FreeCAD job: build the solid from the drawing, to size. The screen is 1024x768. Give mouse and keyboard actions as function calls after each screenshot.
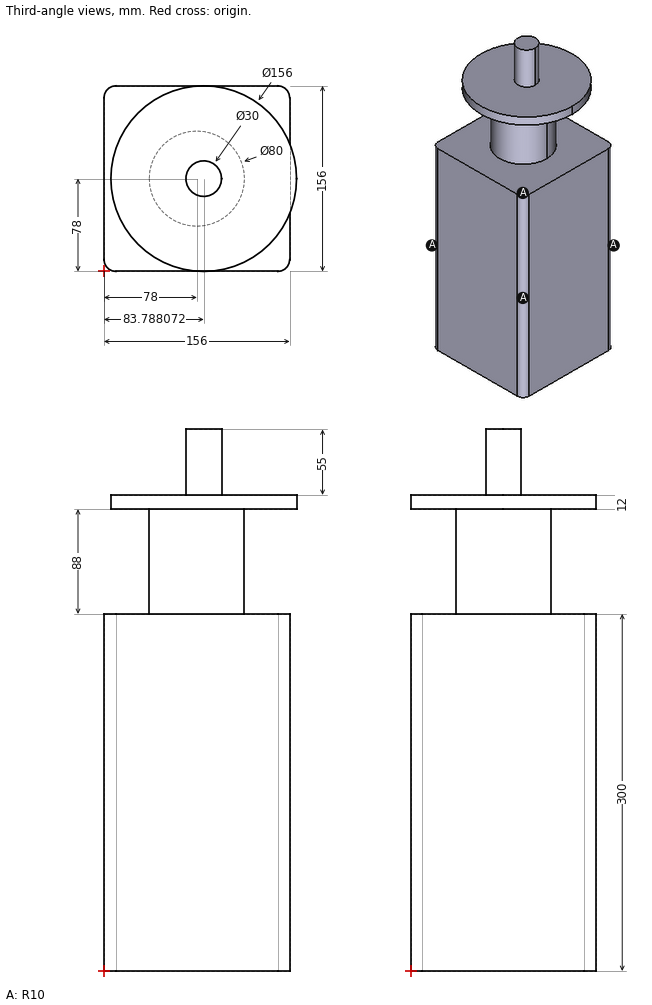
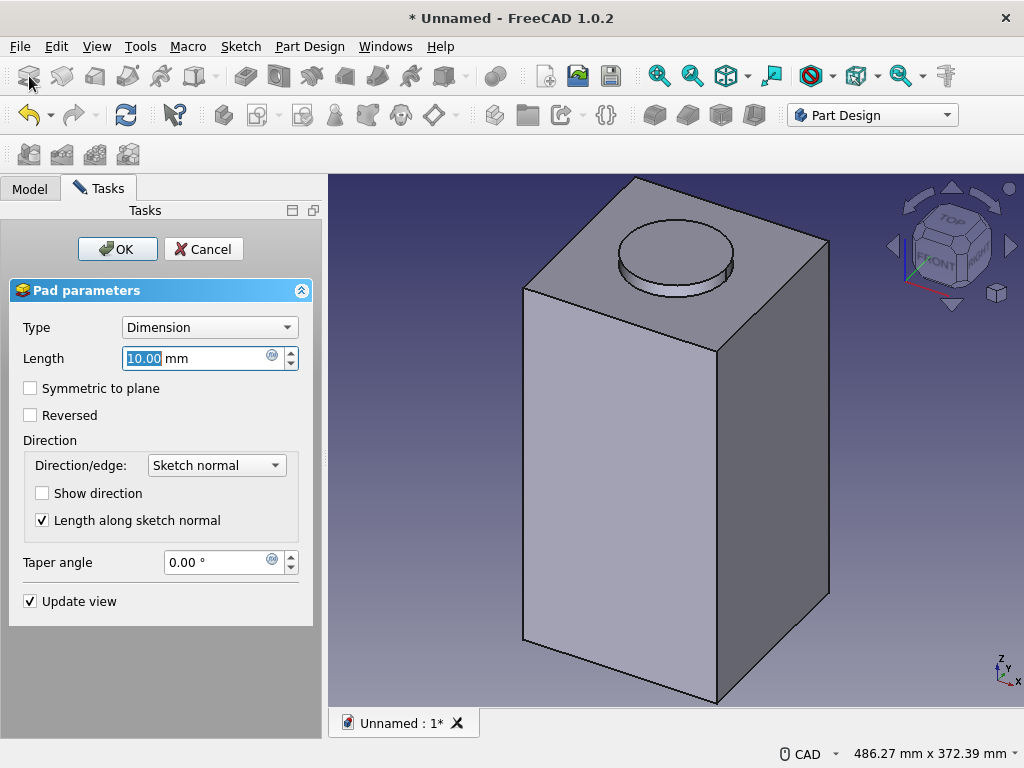
text(88)
key(Tab)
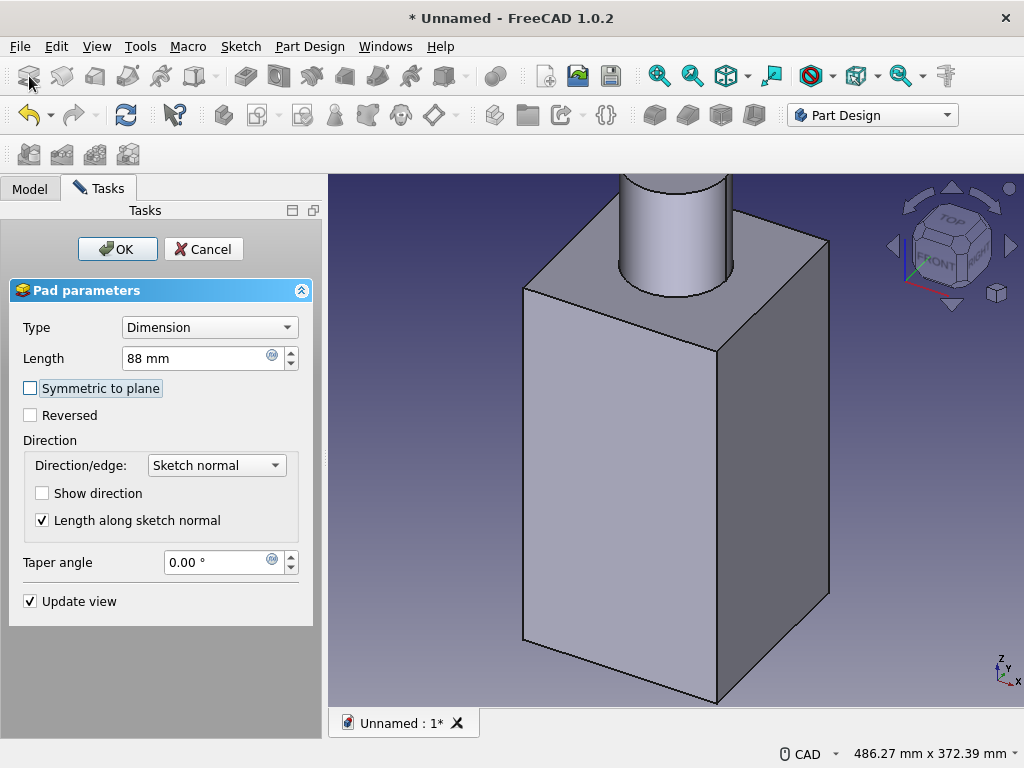
click(118, 249)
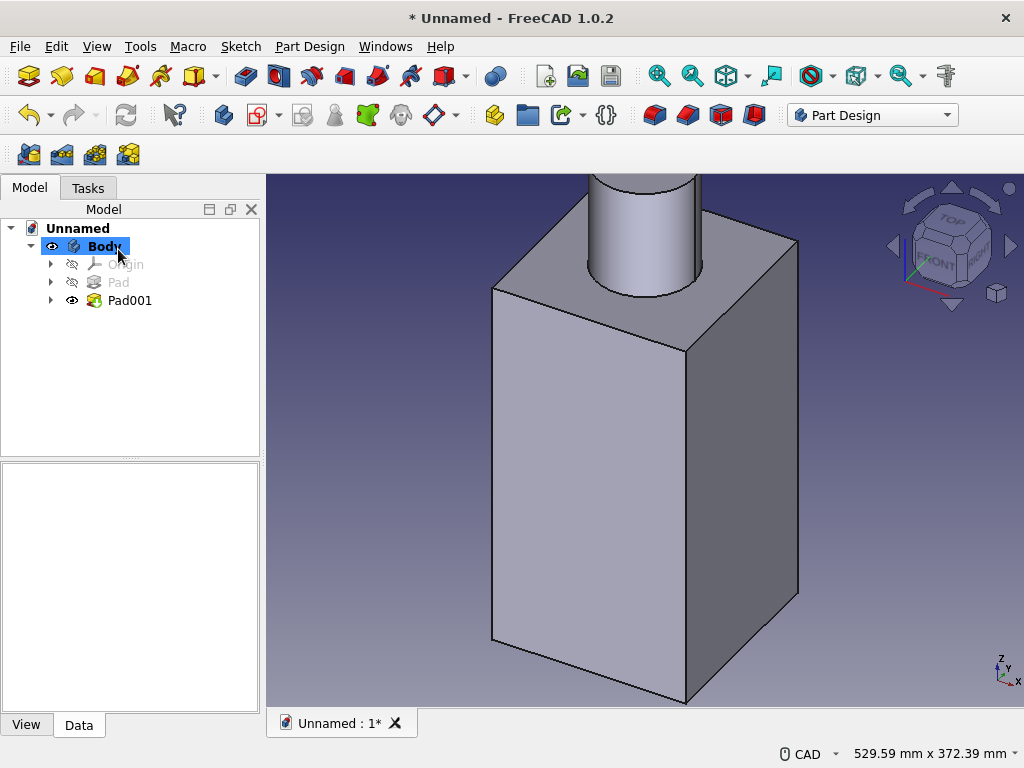
click(660, 76)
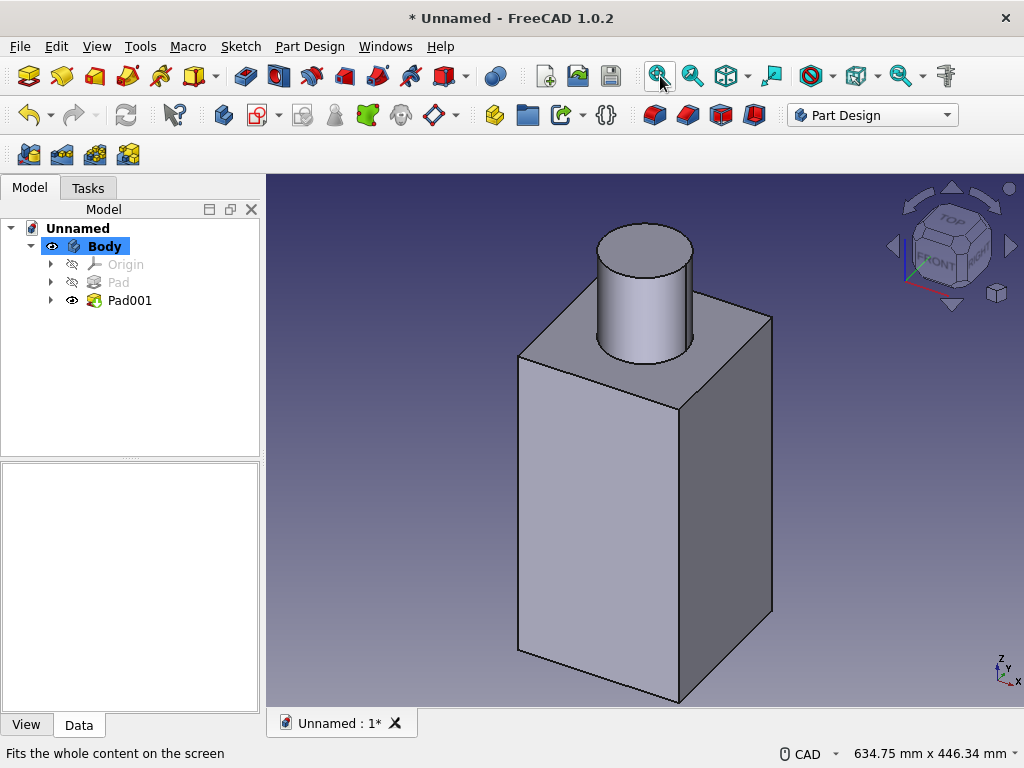
click(645, 250)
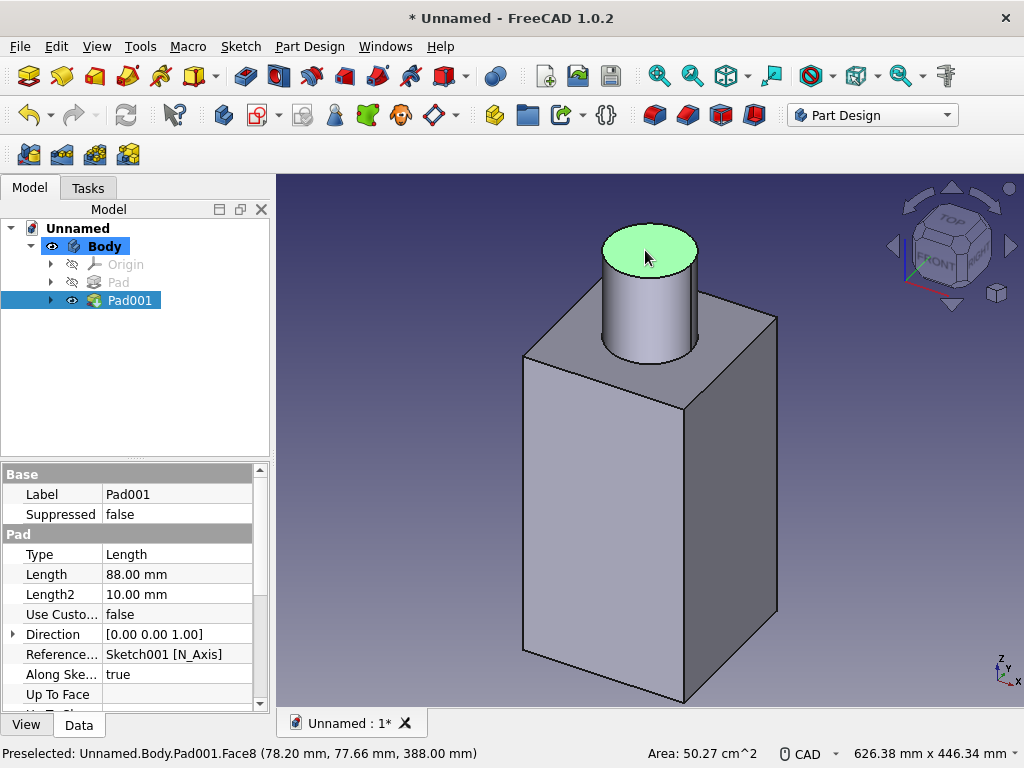
click(256, 116)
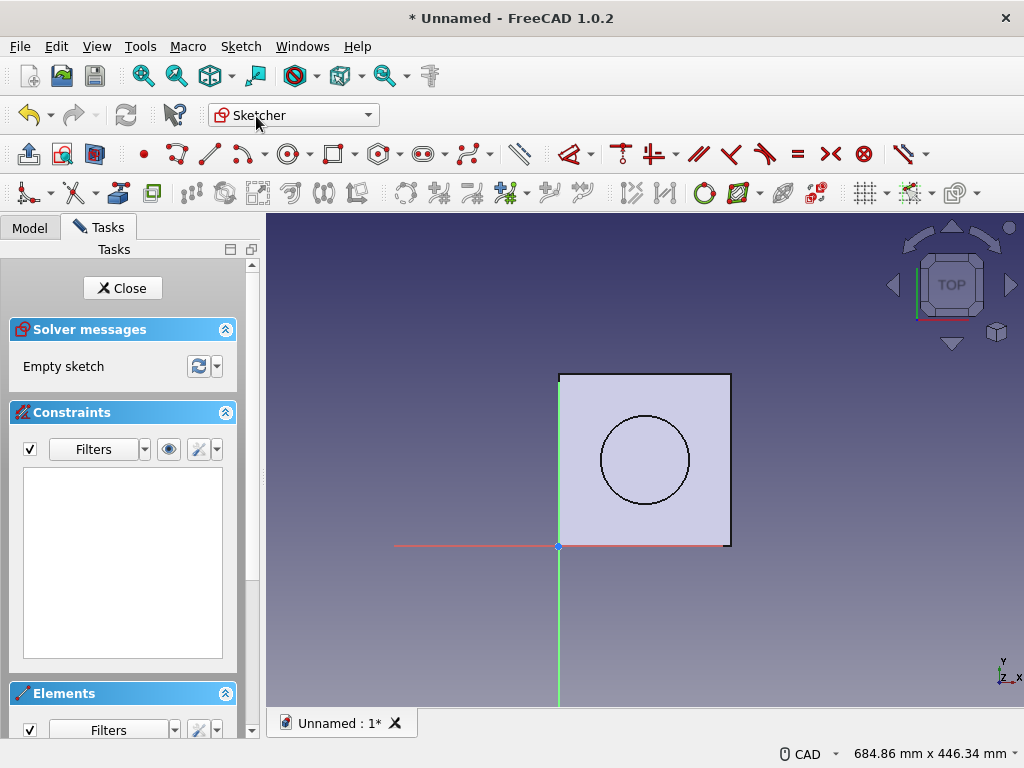
scroll(735, 460, up, 3)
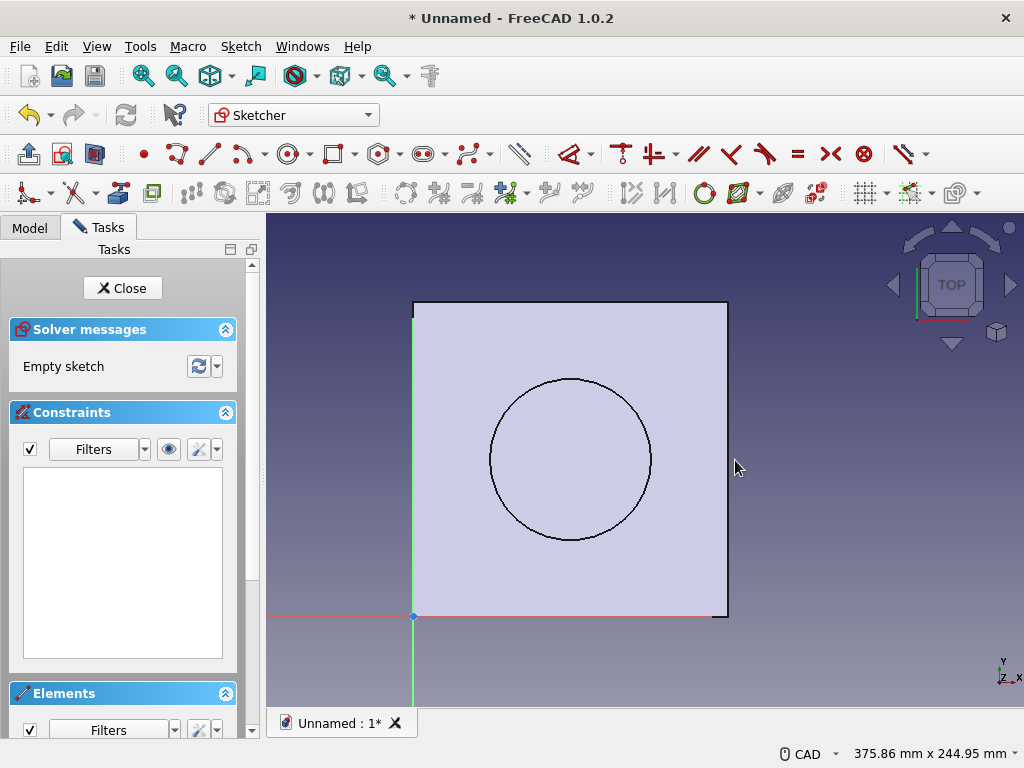
click(288, 154)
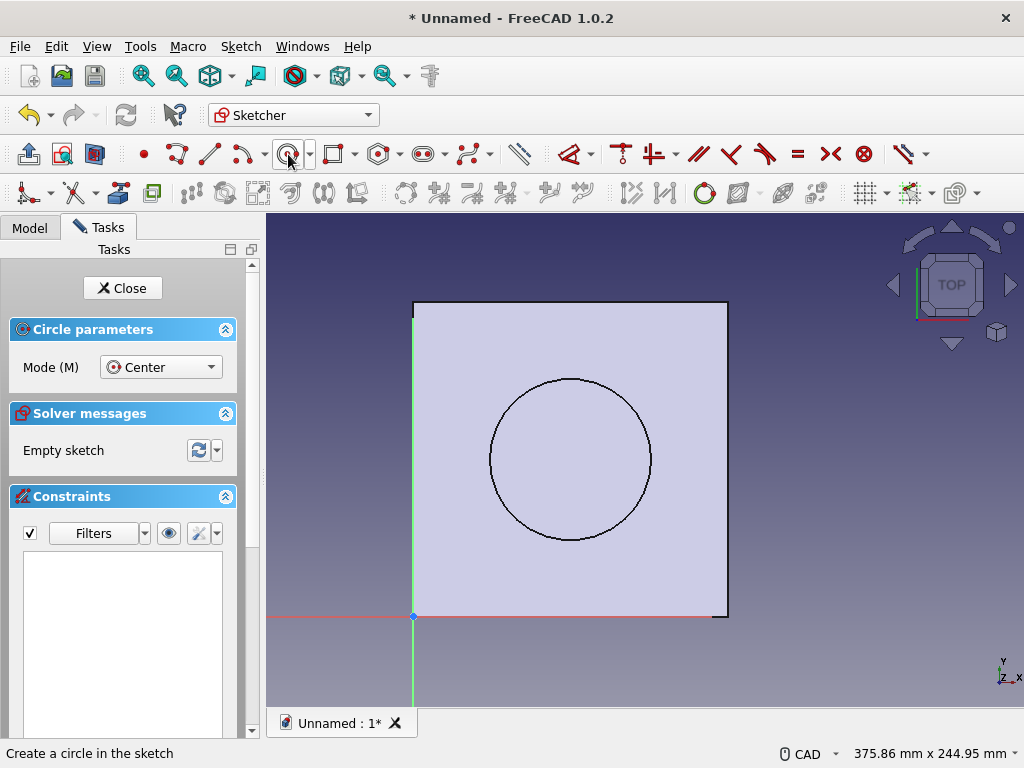
click(582, 460)
move(693, 348)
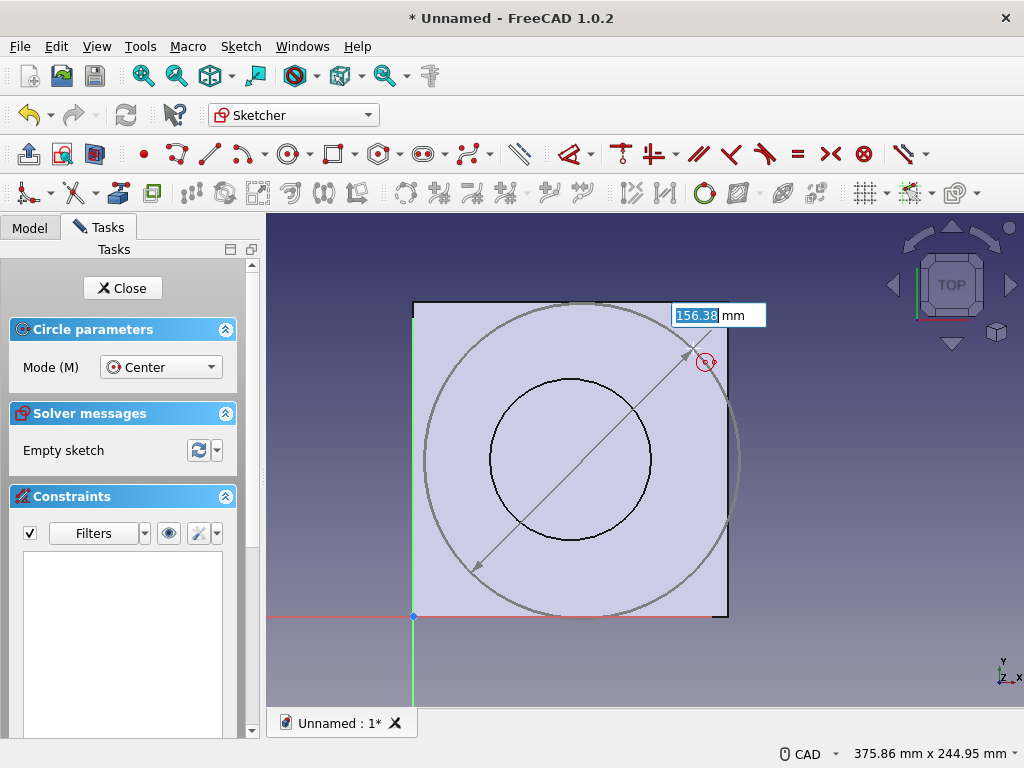
text(156)
key(Return)
key(Escape)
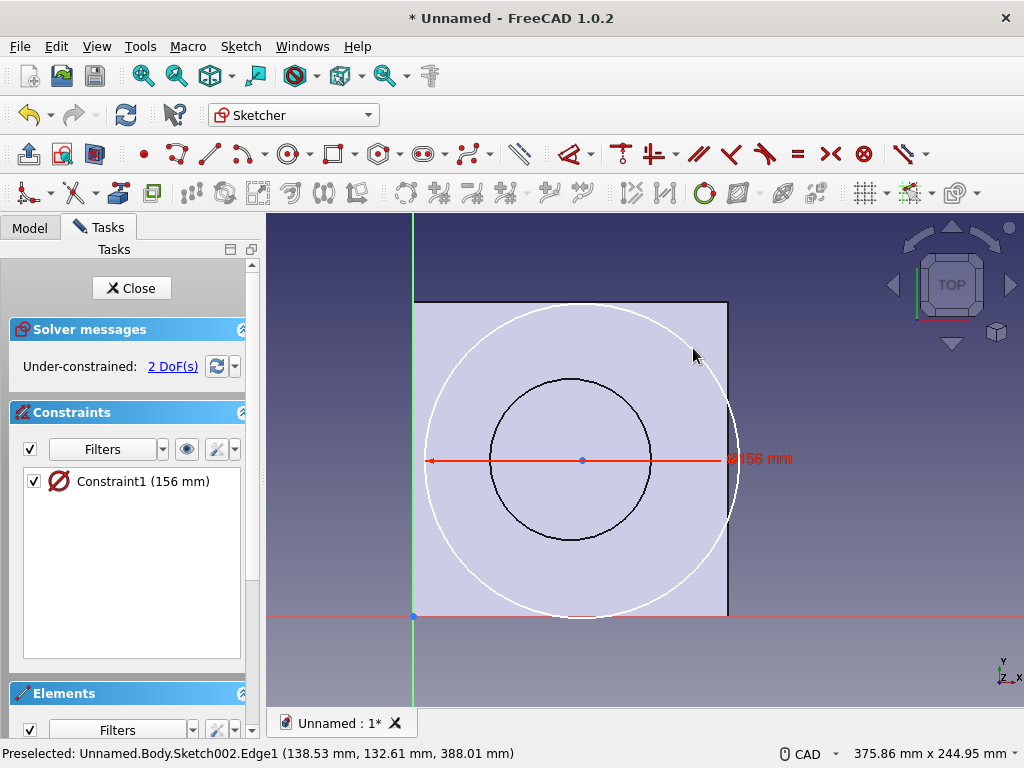
click(568, 154)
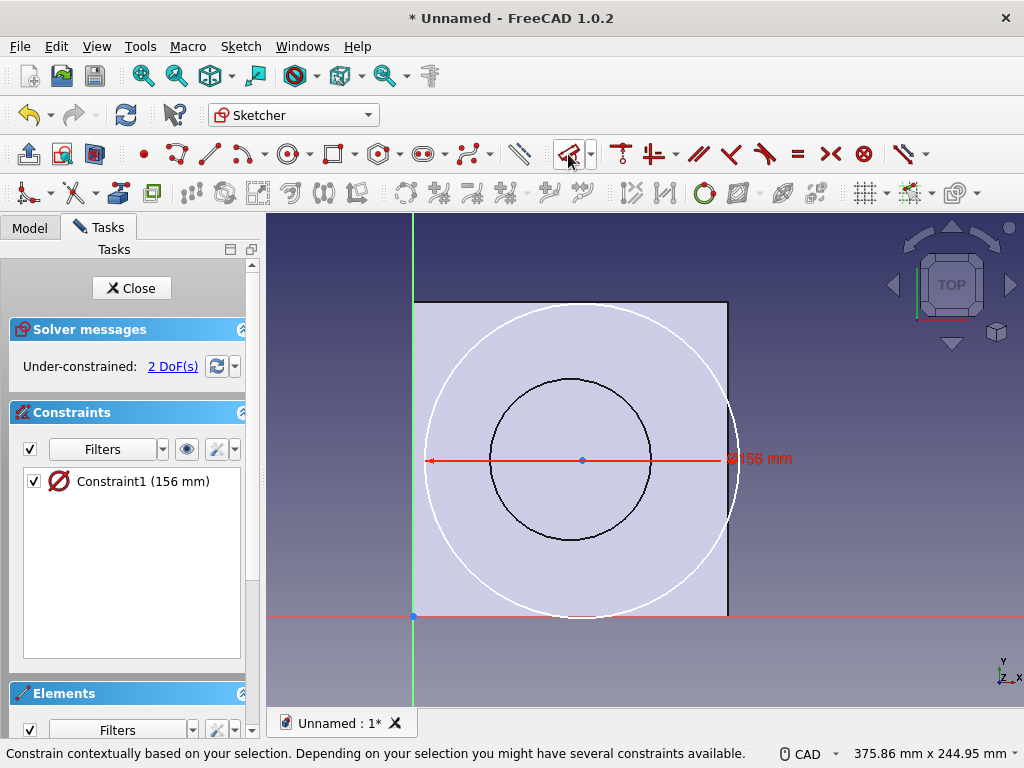
click(582, 461)
click(379, 539)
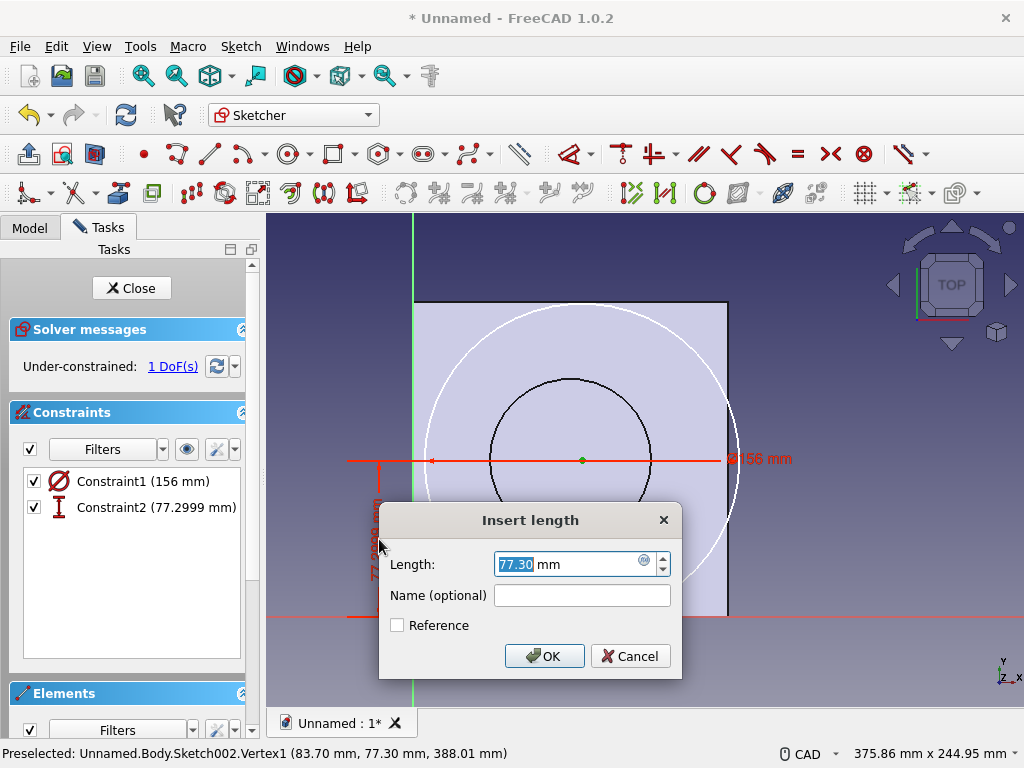
text(78)
key(Return)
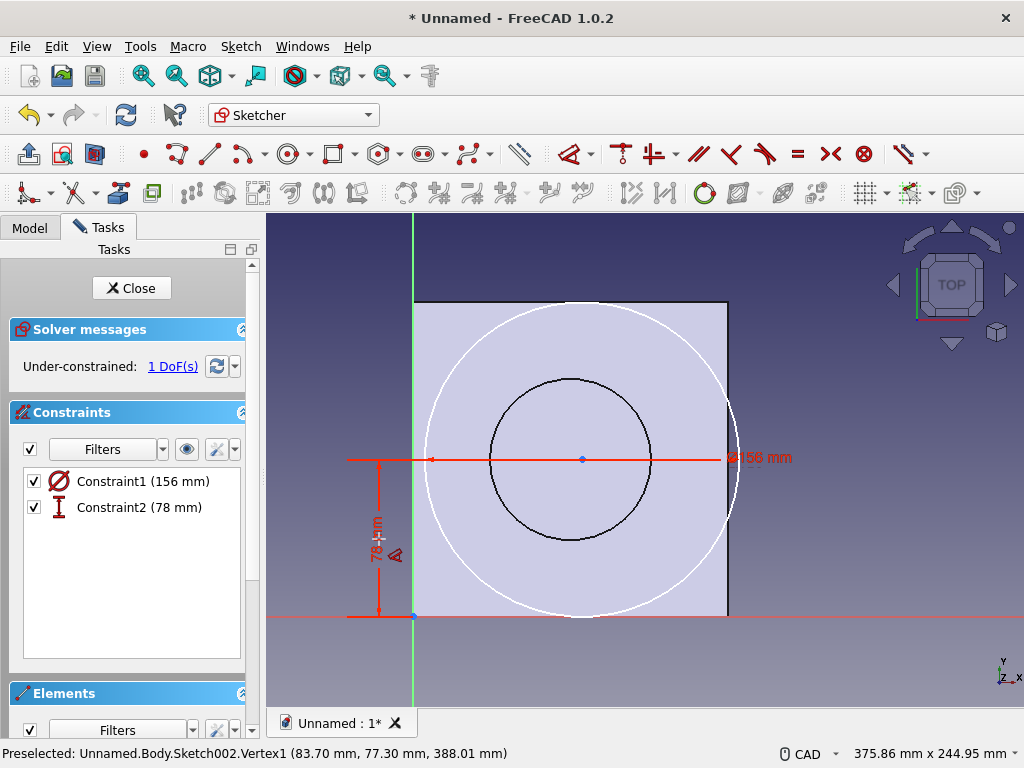
click(582, 460)
click(498, 651)